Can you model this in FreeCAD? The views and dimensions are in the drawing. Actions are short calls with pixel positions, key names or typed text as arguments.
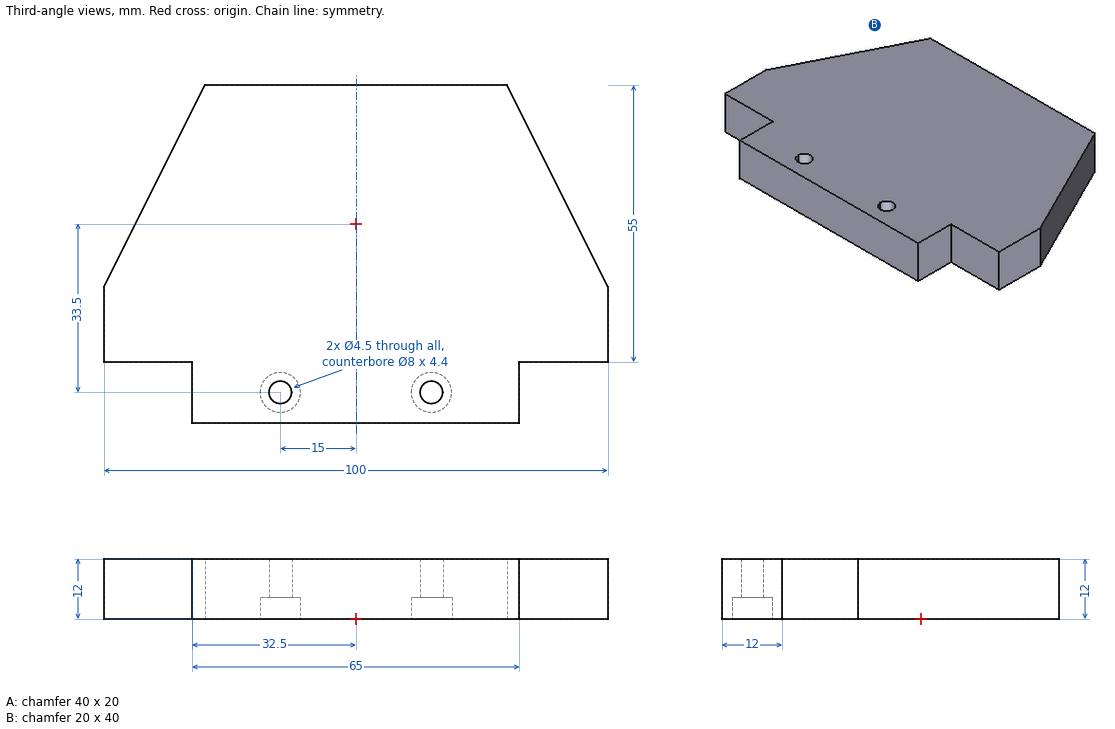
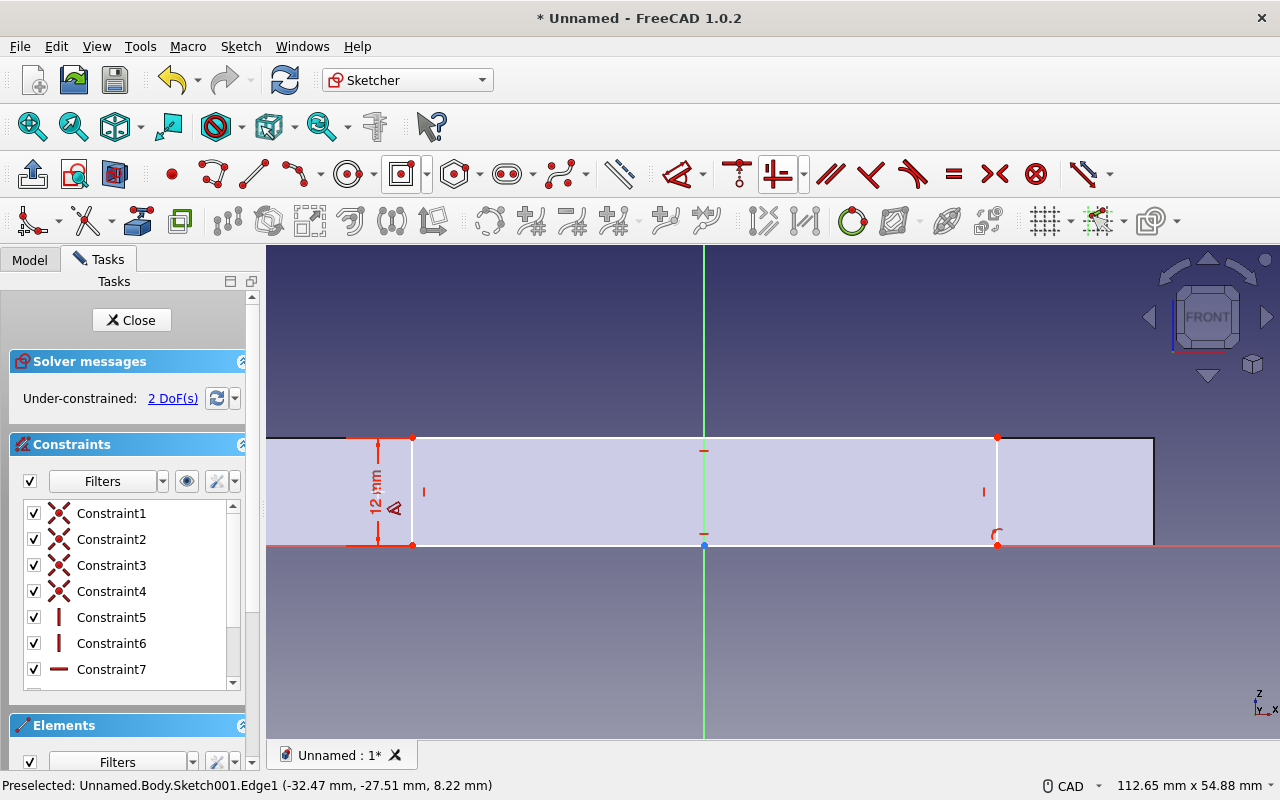
click(587, 546)
click(570, 580)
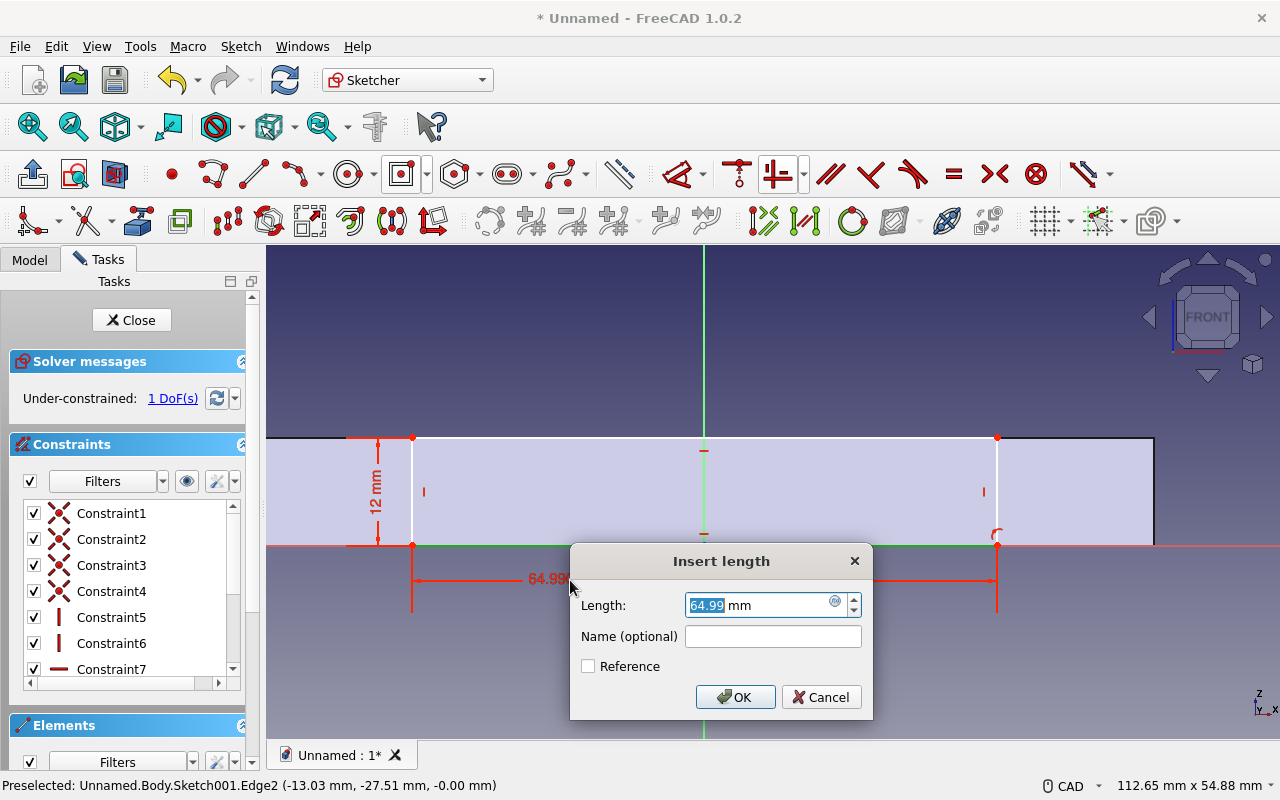
text(65)
key(Return)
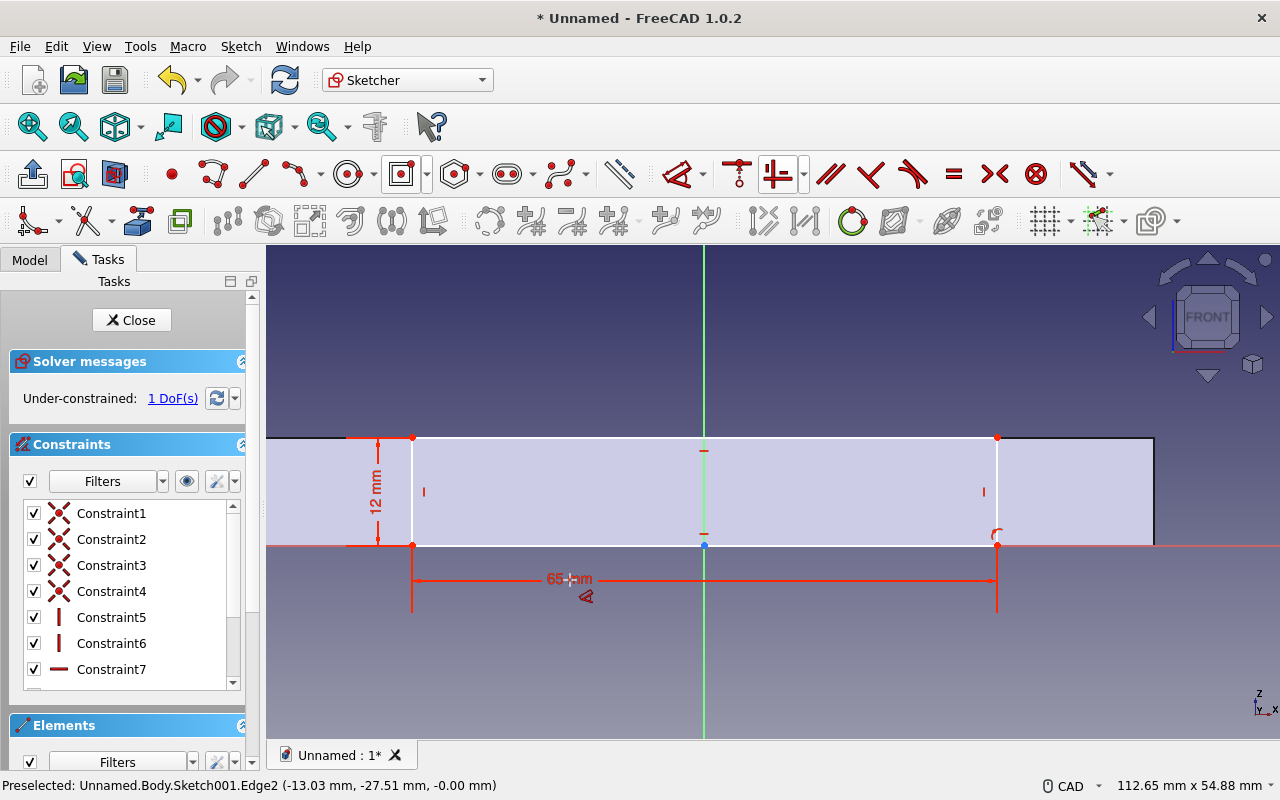
click(412, 438)
click(491, 580)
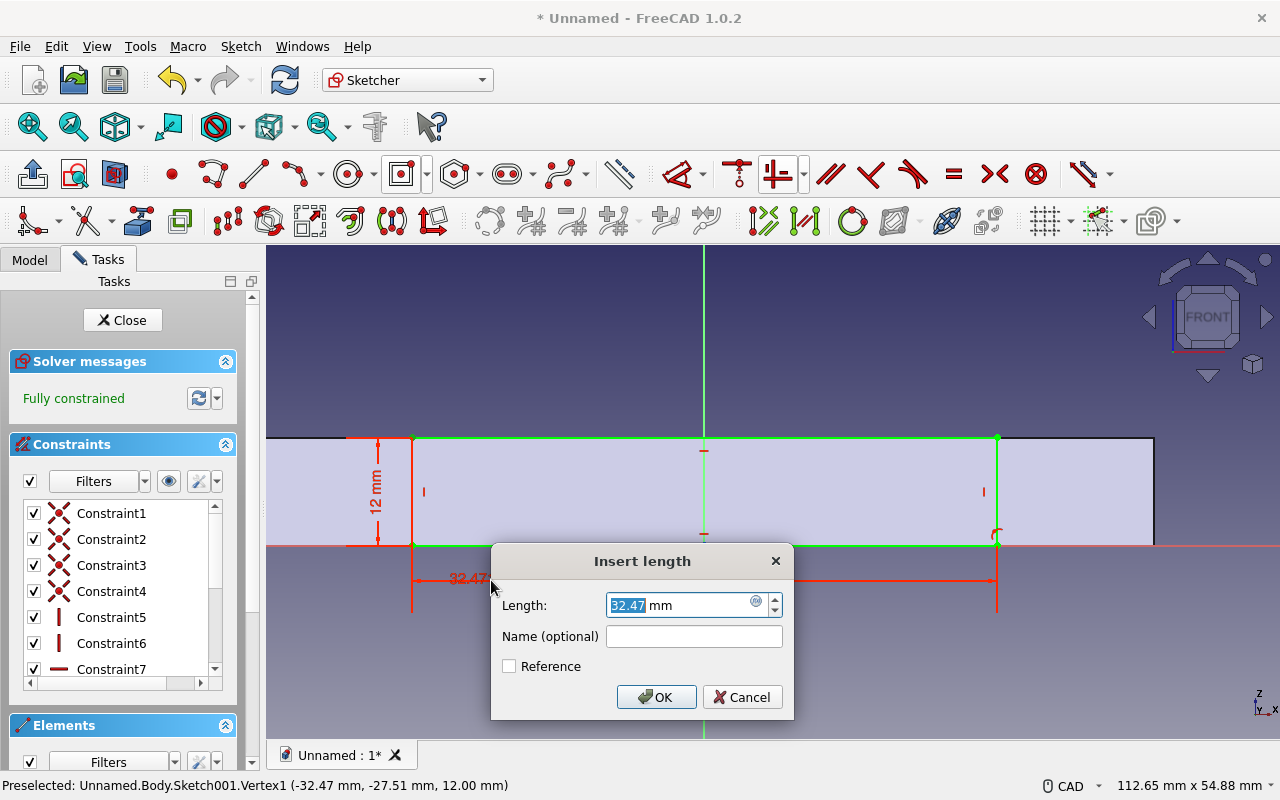
text(32.5)
key(Return)
key(Escape)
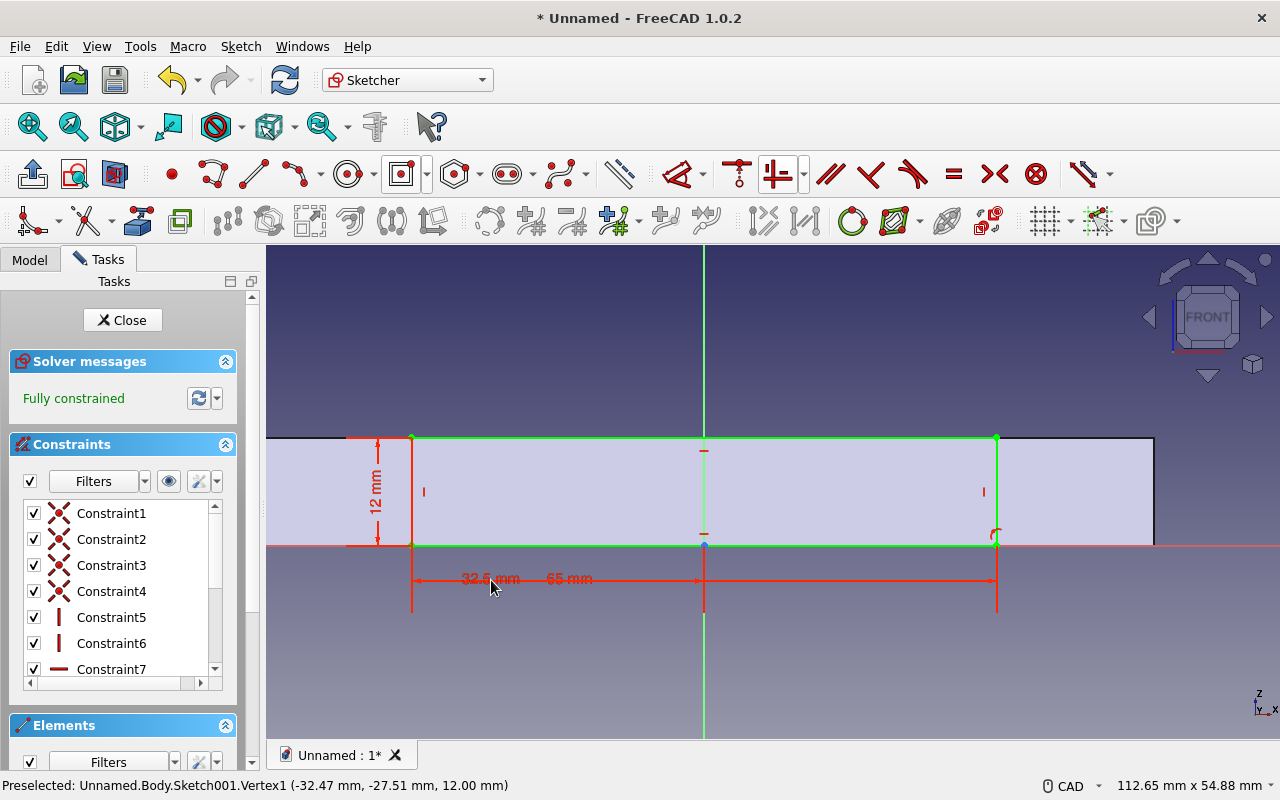
click(123, 320)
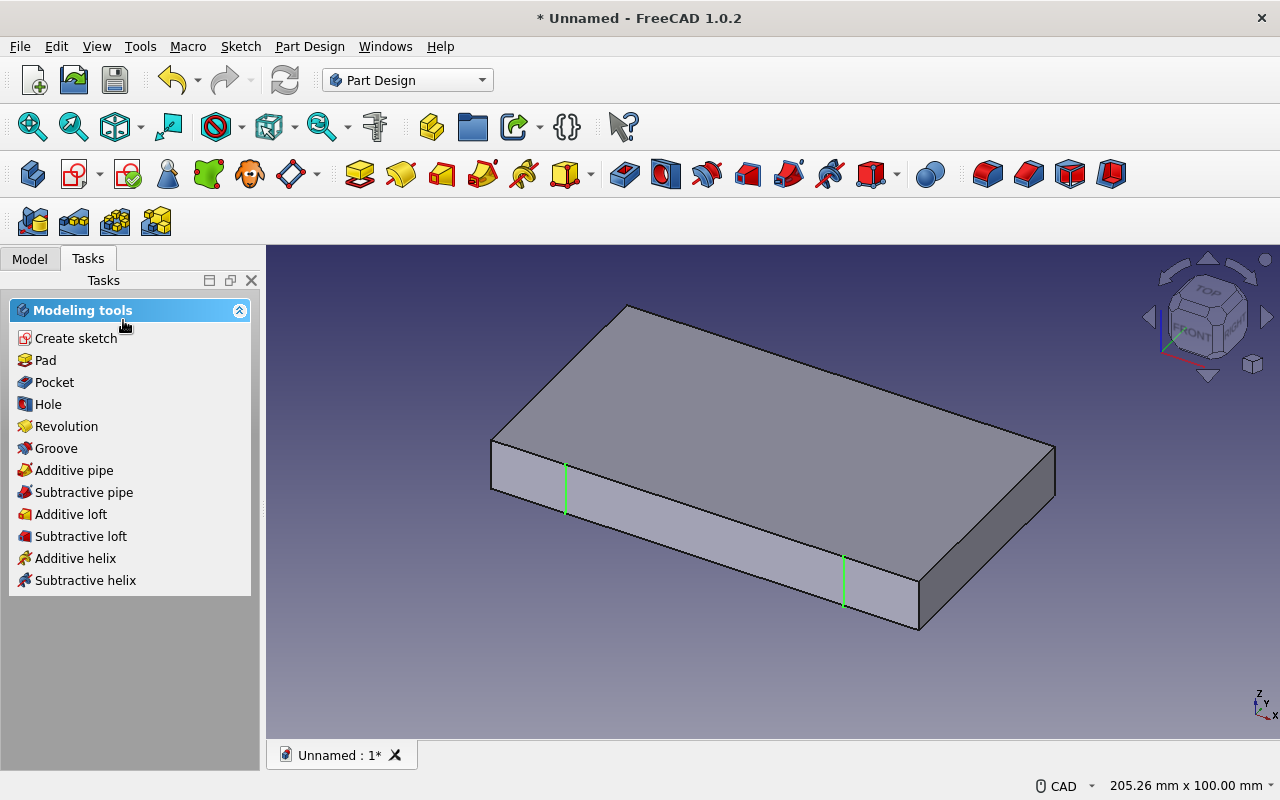
click(360, 174)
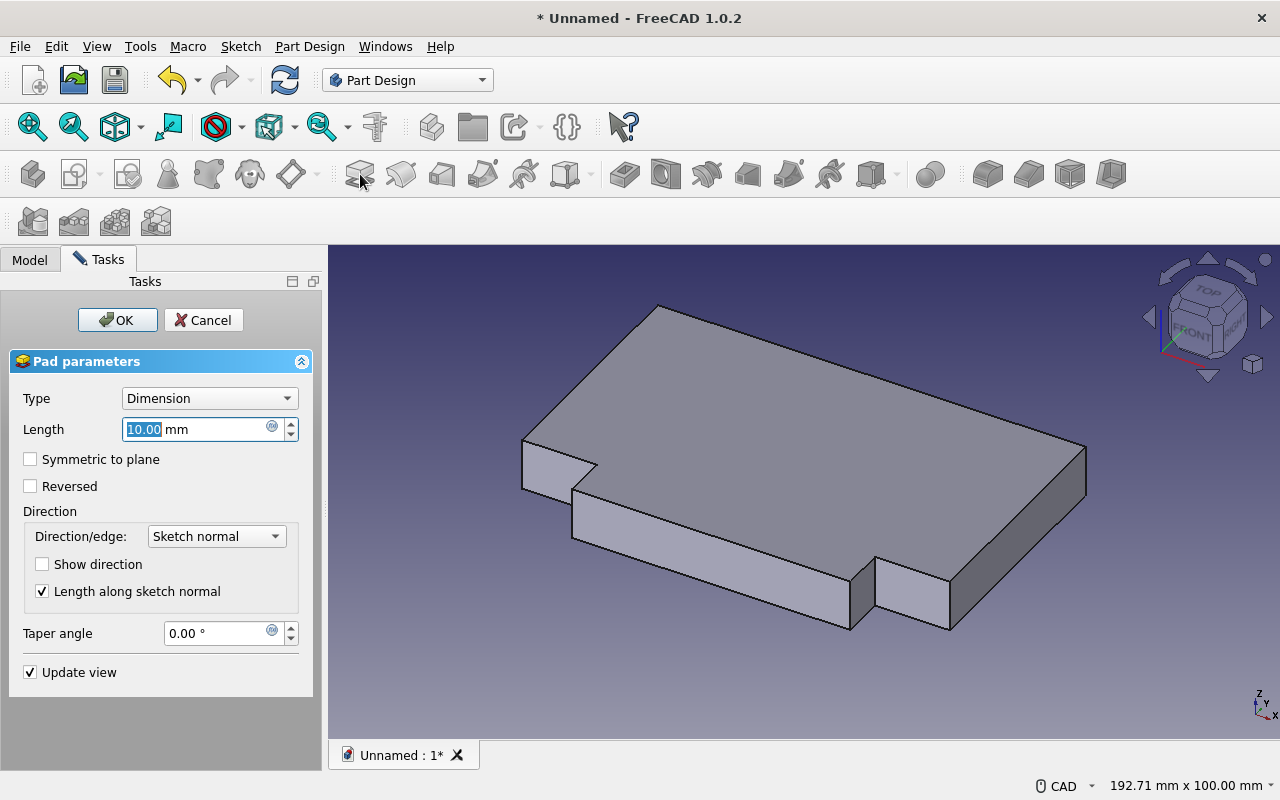
text(12)
key(Tab)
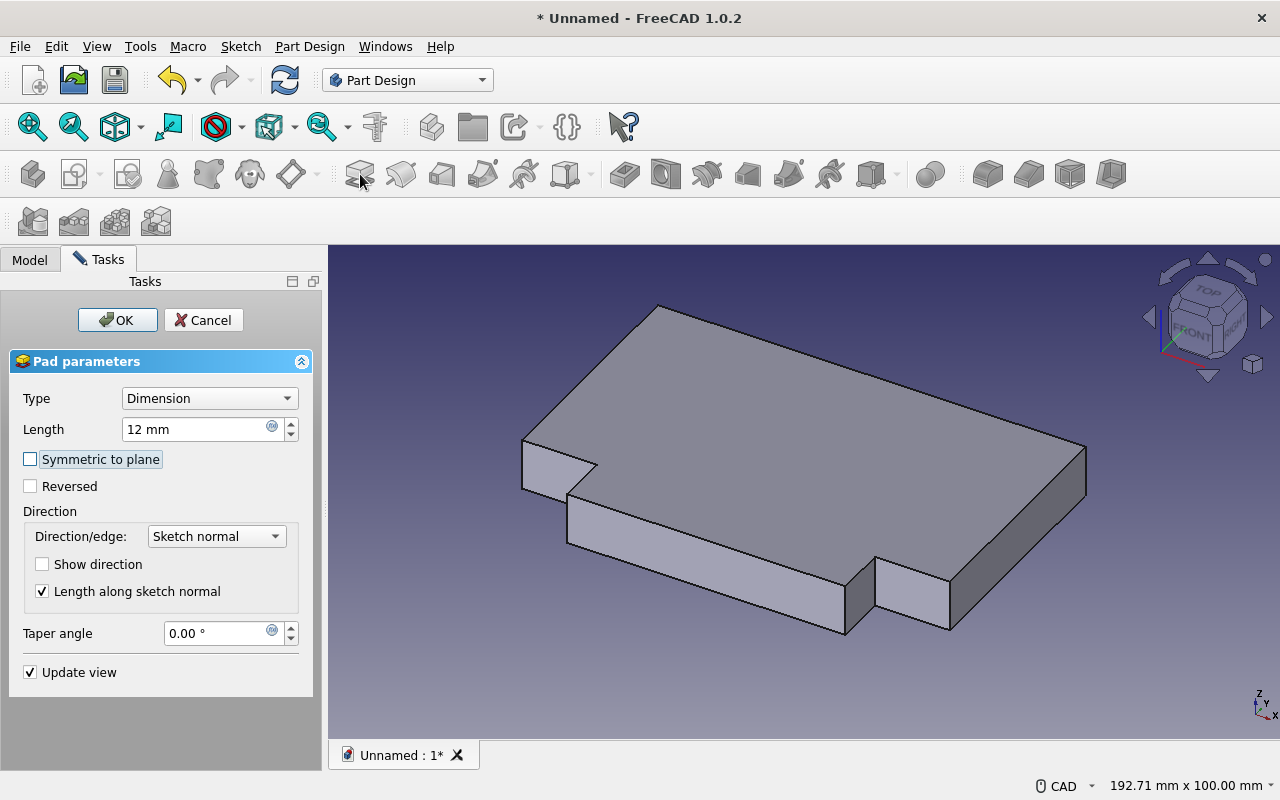
click(118, 320)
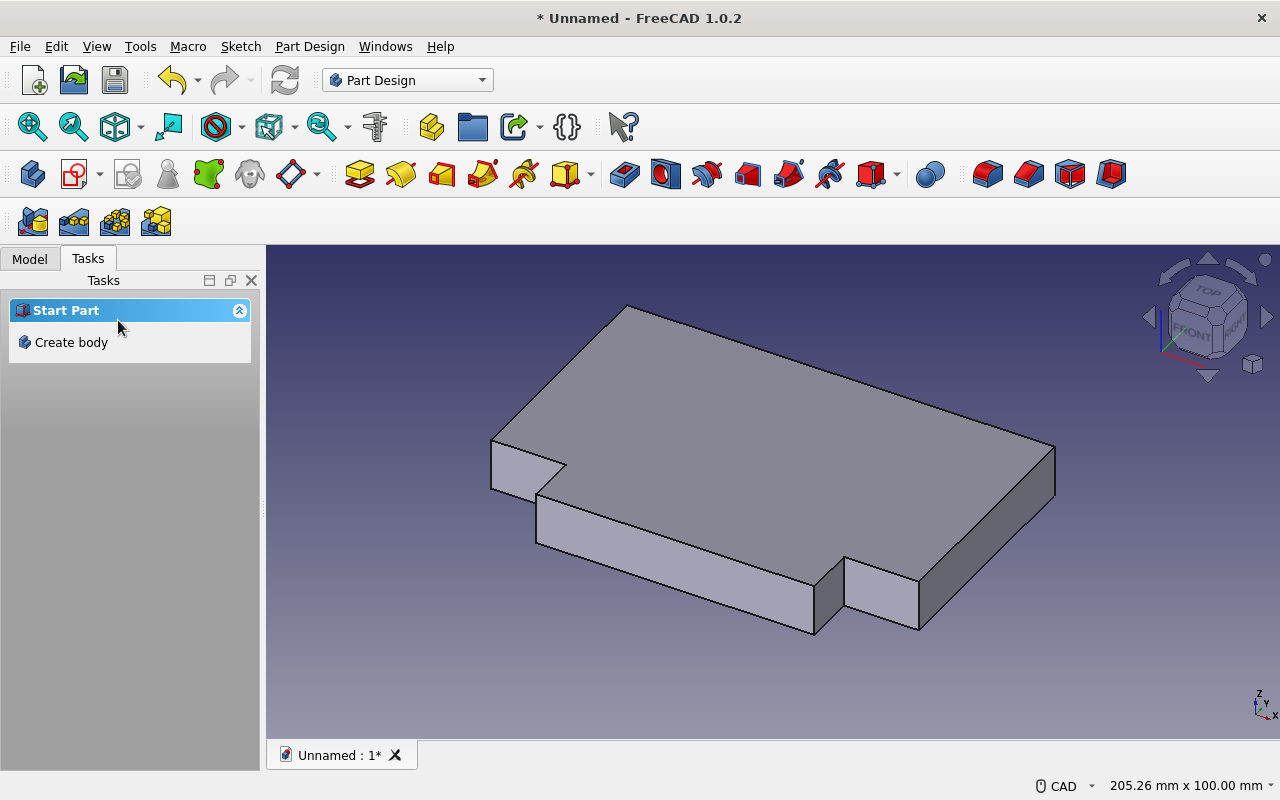
key(5)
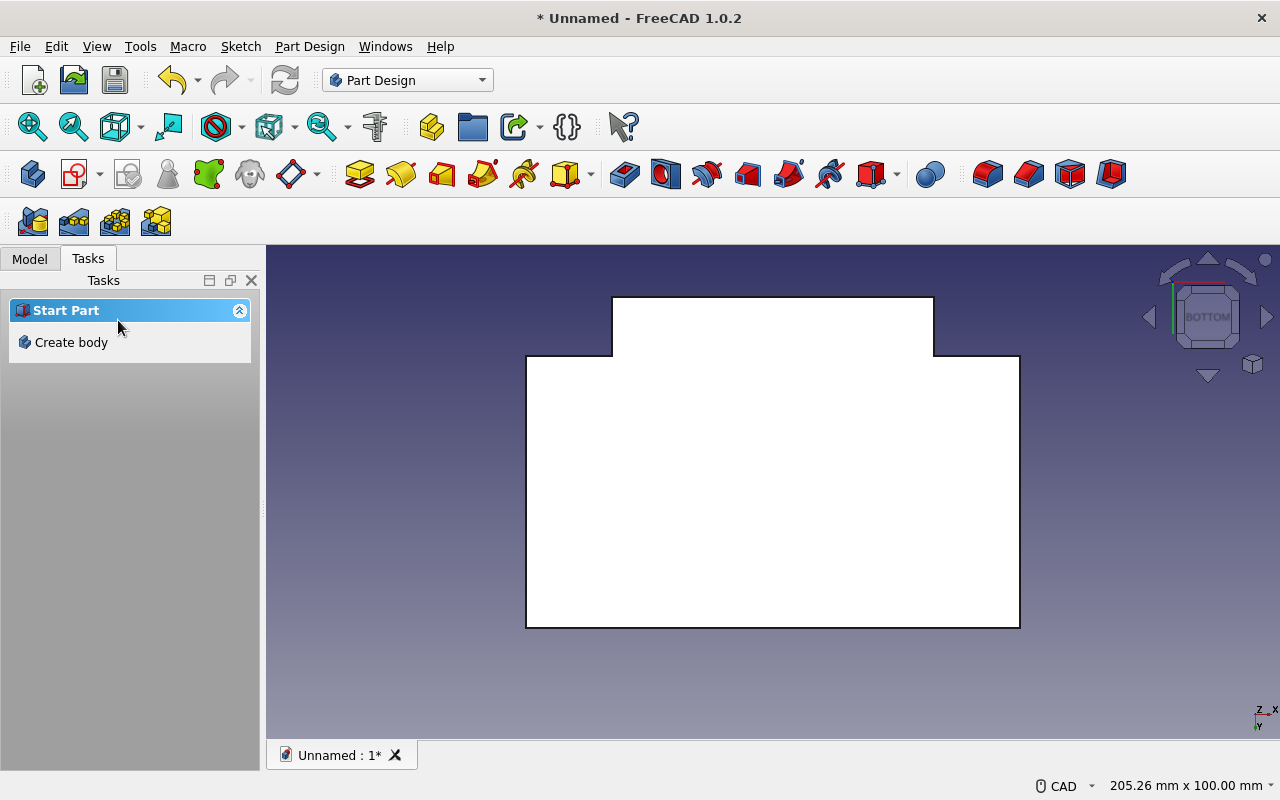
click(773, 461)